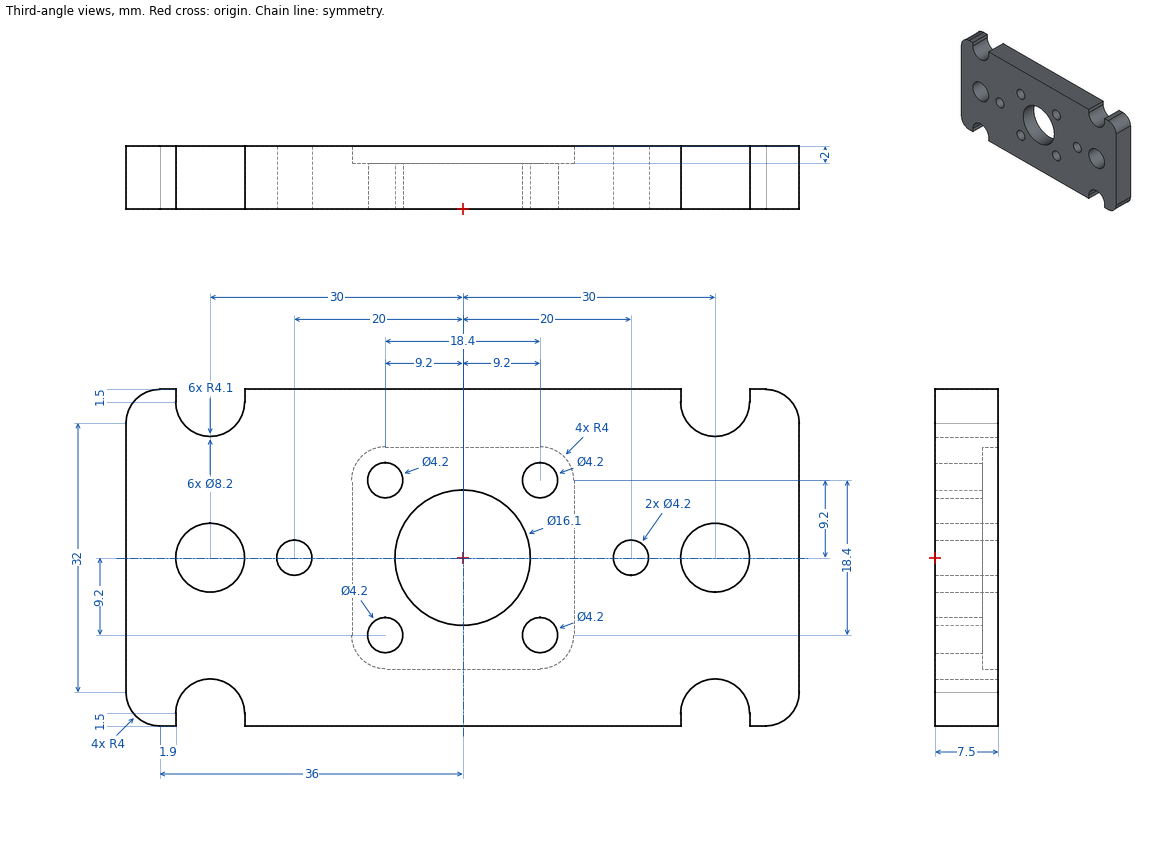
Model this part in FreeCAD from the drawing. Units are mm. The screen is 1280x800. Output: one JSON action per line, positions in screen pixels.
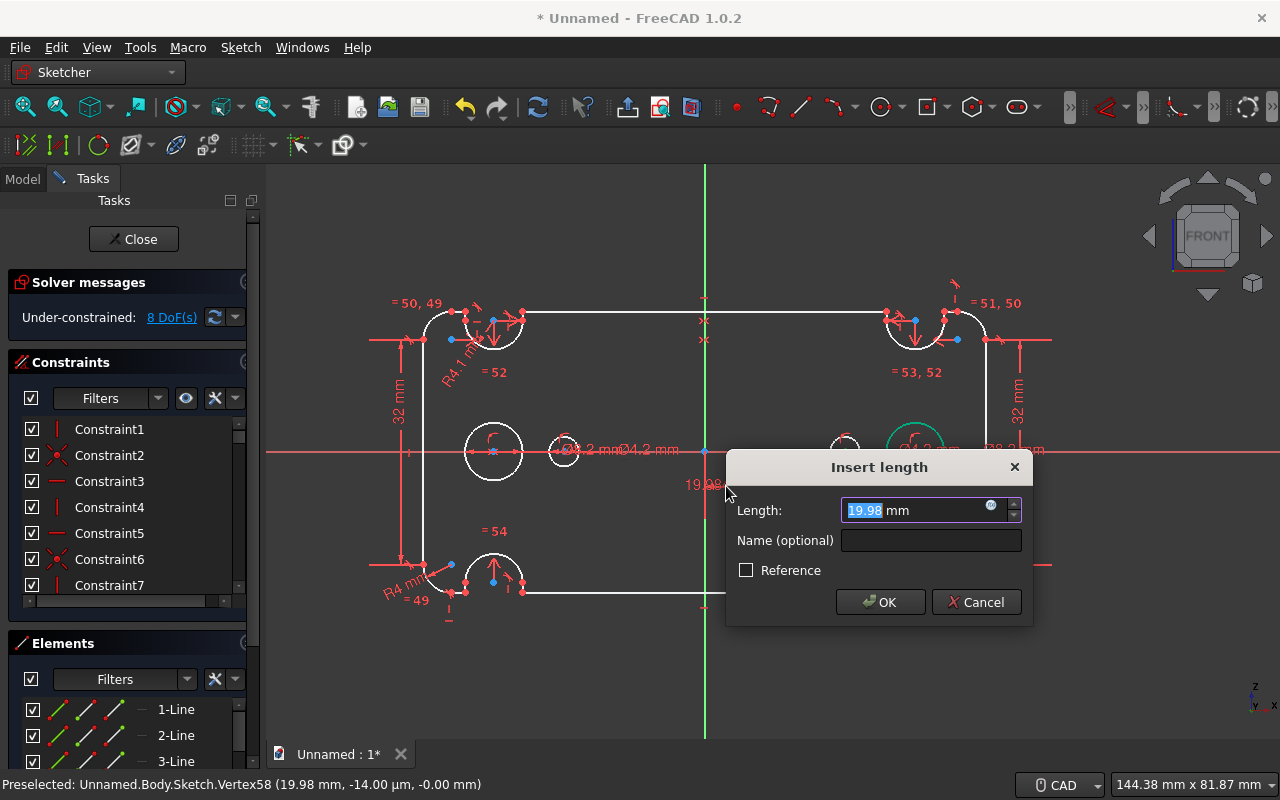
{"action": "type", "text": "20"}
{"action": "key", "text": "Return"}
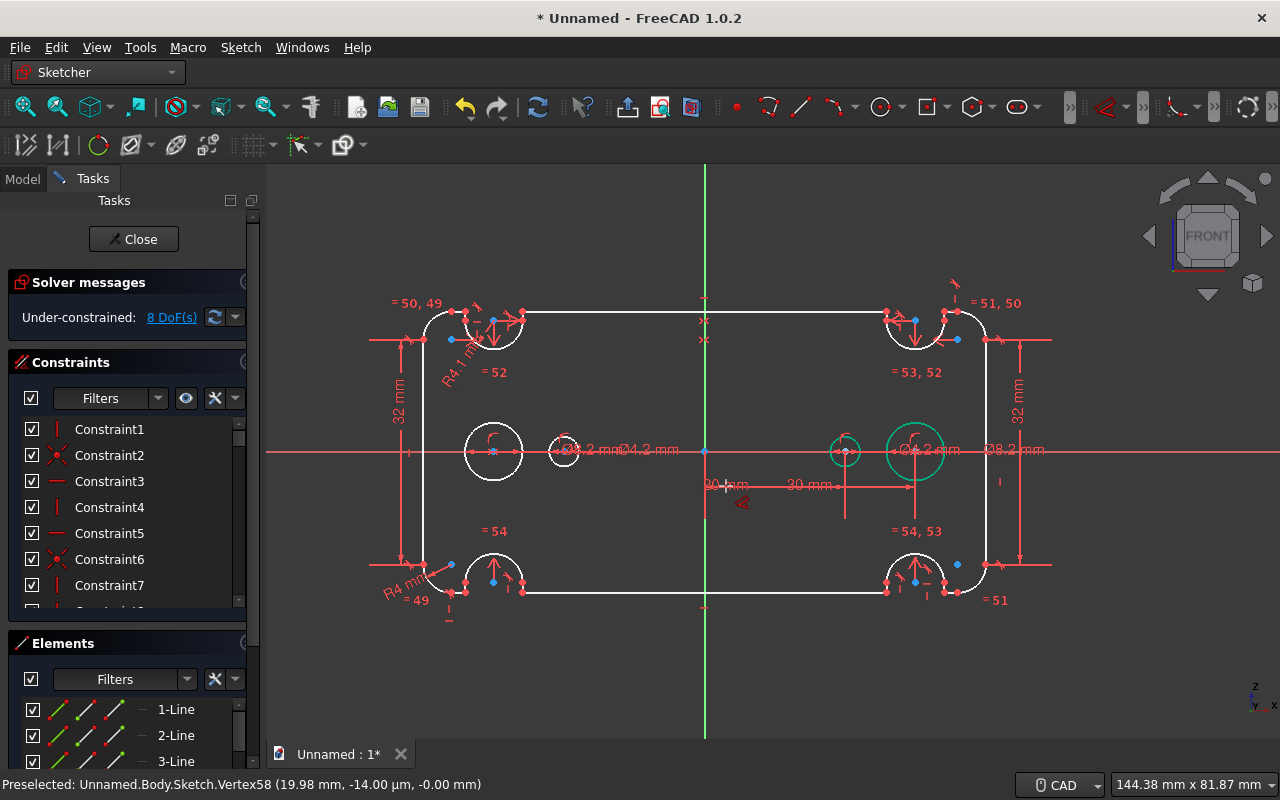
{"action": "left_click", "coordinate": [564, 452]}
{"action": "left_click", "coordinate": [634, 486]}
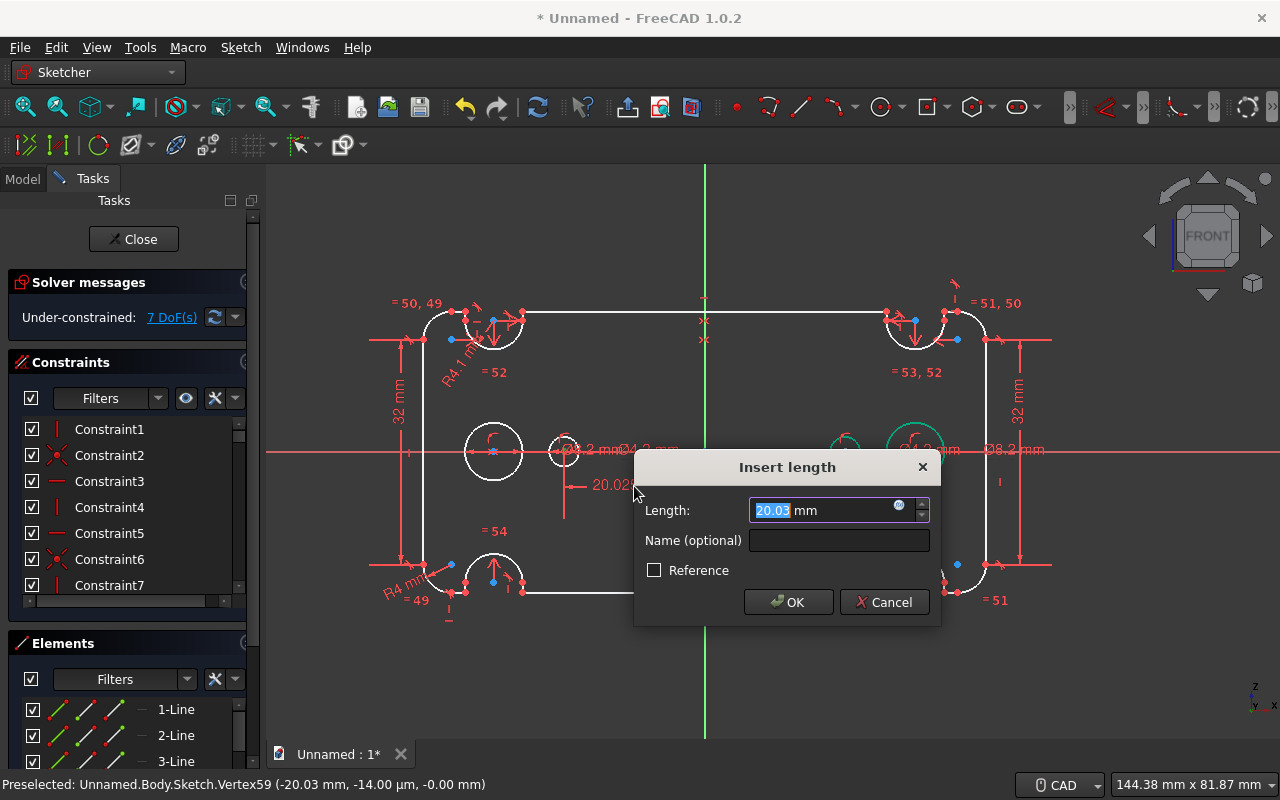
{"action": "type", "text": "20"}
{"action": "key", "text": "Return"}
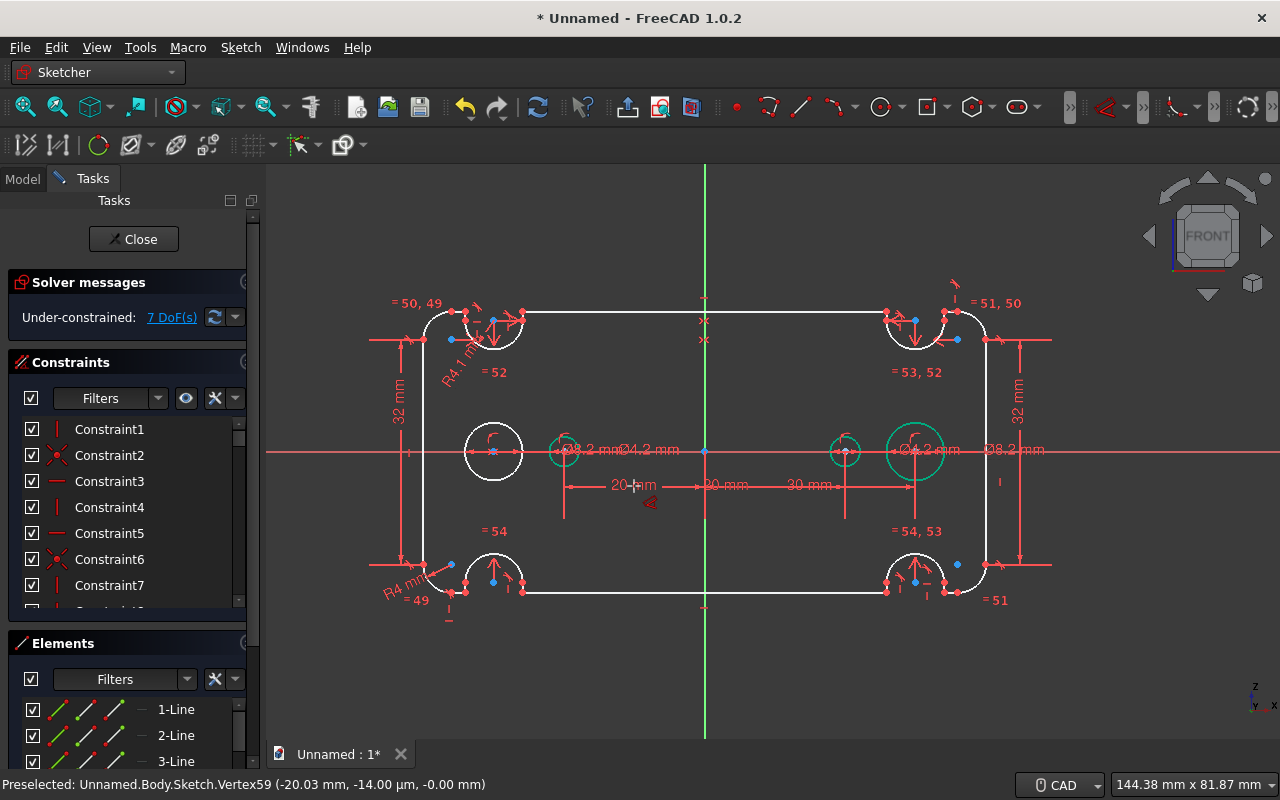
{"action": "left_click", "coordinate": [494, 452]}
{"action": "left_click", "coordinate": [551, 486]}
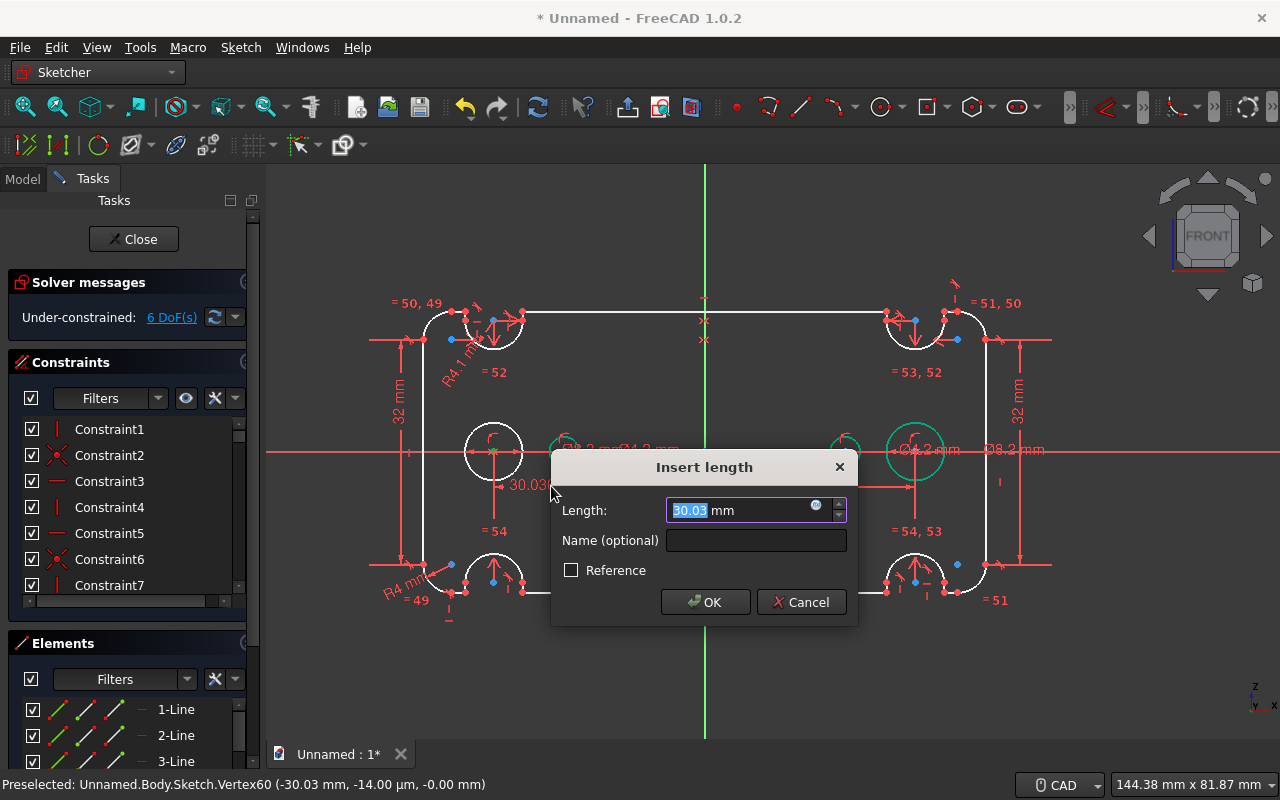
{"action": "type", "text": "30"}
{"action": "key", "text": "Return"}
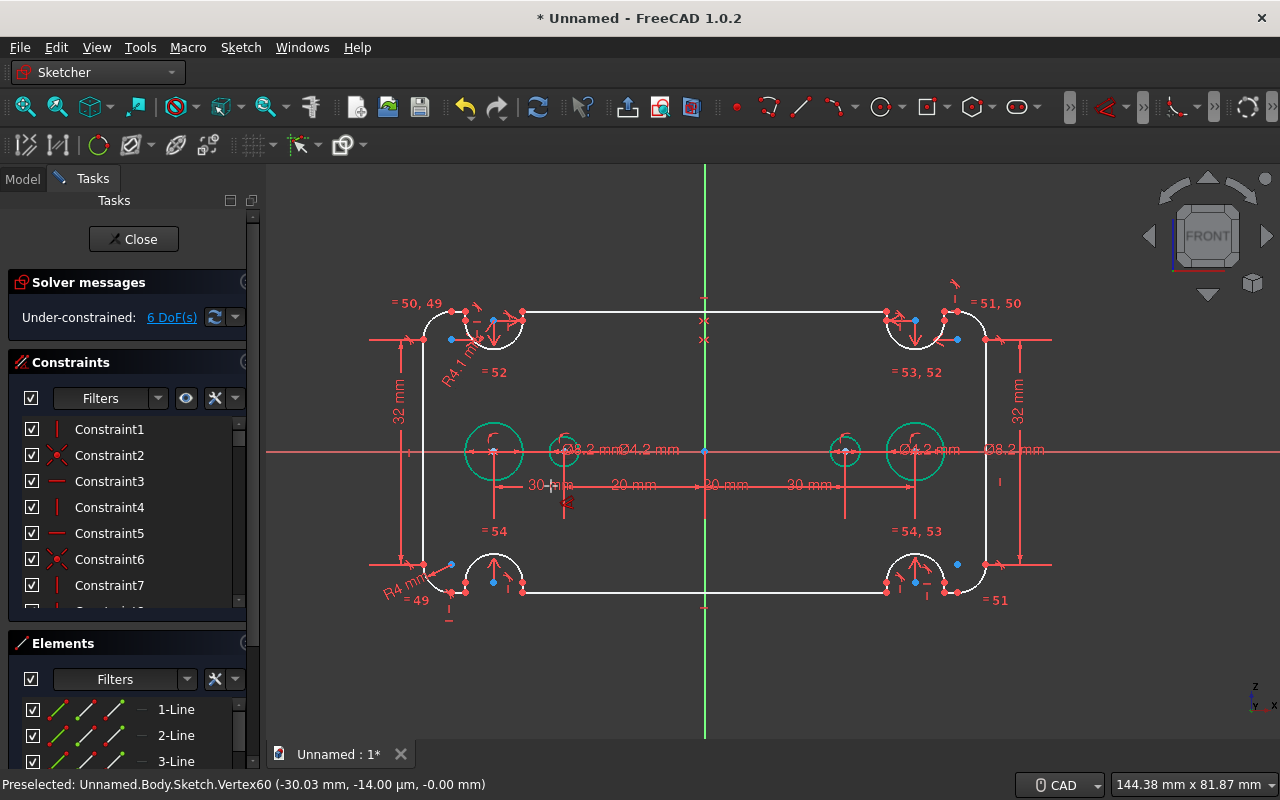
{"action": "scroll", "coordinate": [465, 588], "scroll_direction": "up", "scroll_amount": 7}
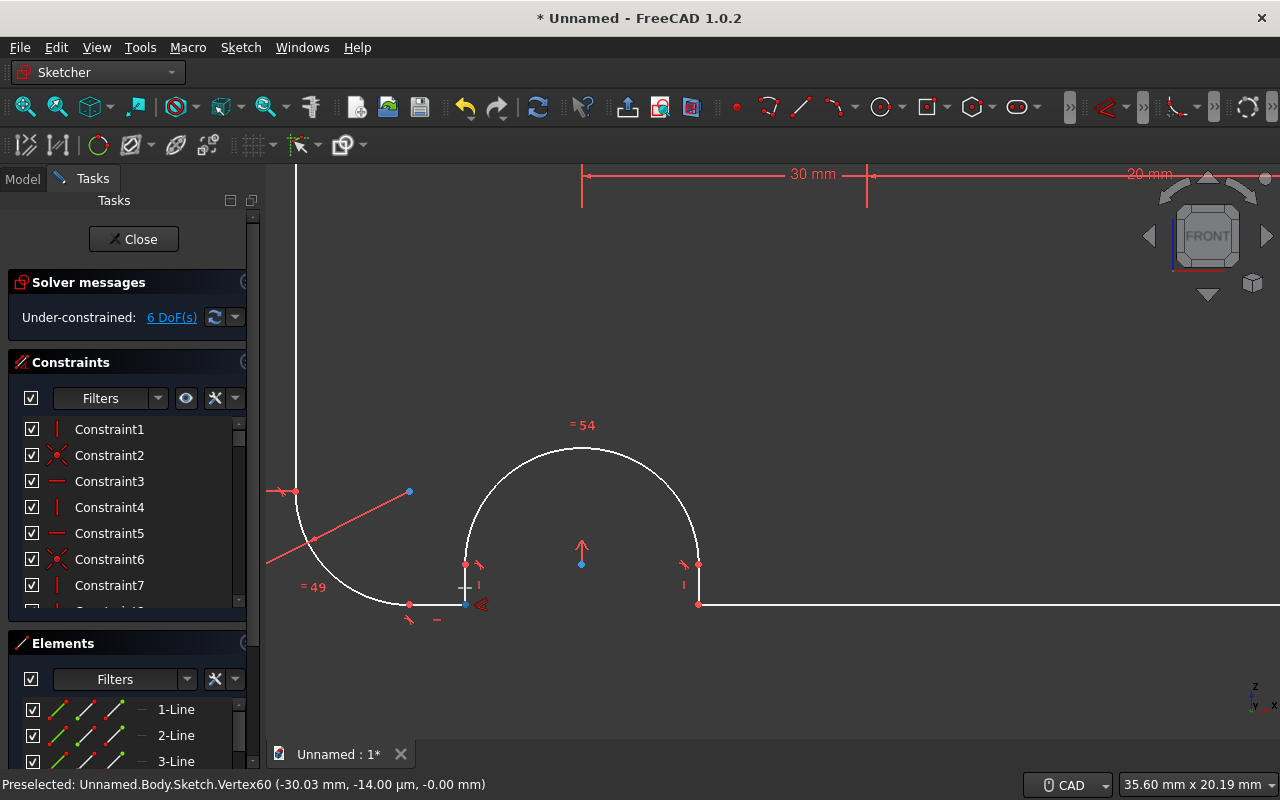
{"action": "left_click", "coordinate": [465, 585]}
{"action": "left_click", "coordinate": [431, 585]}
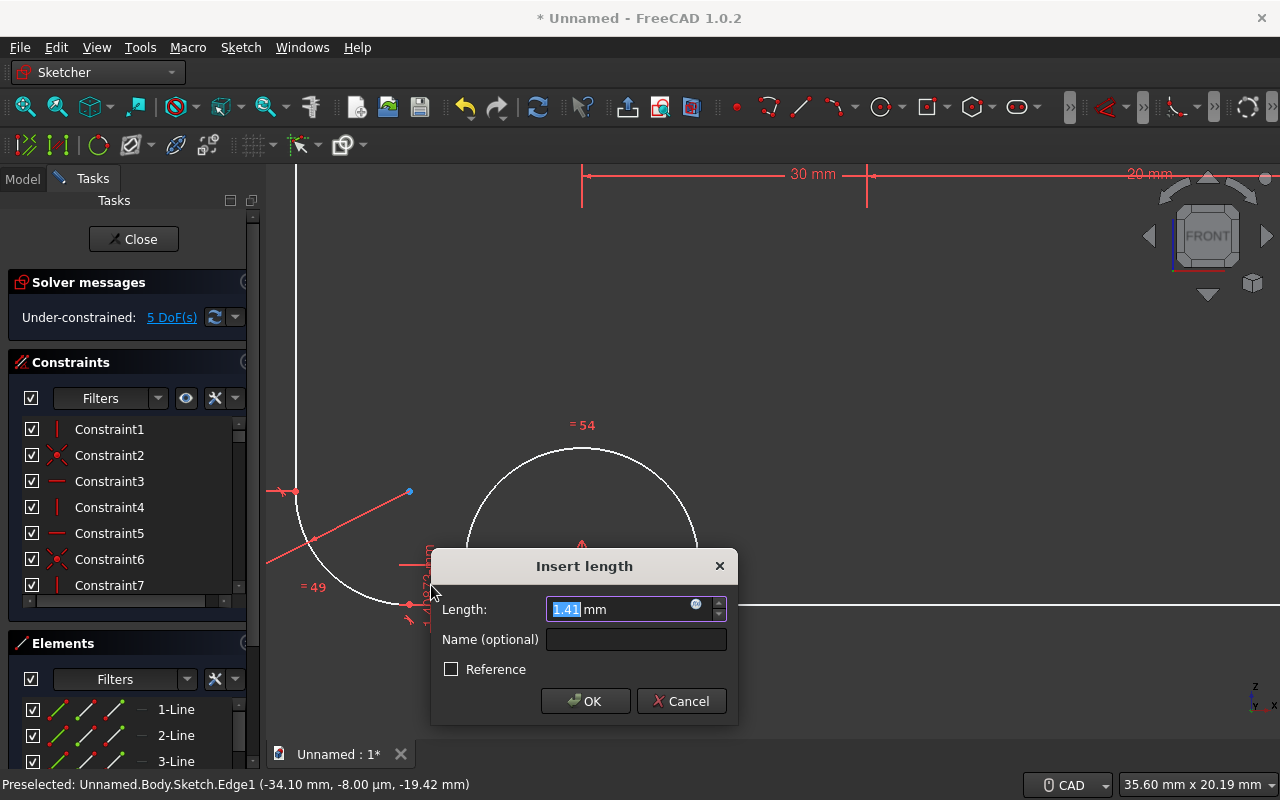
{"action": "type", "text": "1.5"}
{"action": "key", "text": "Return"}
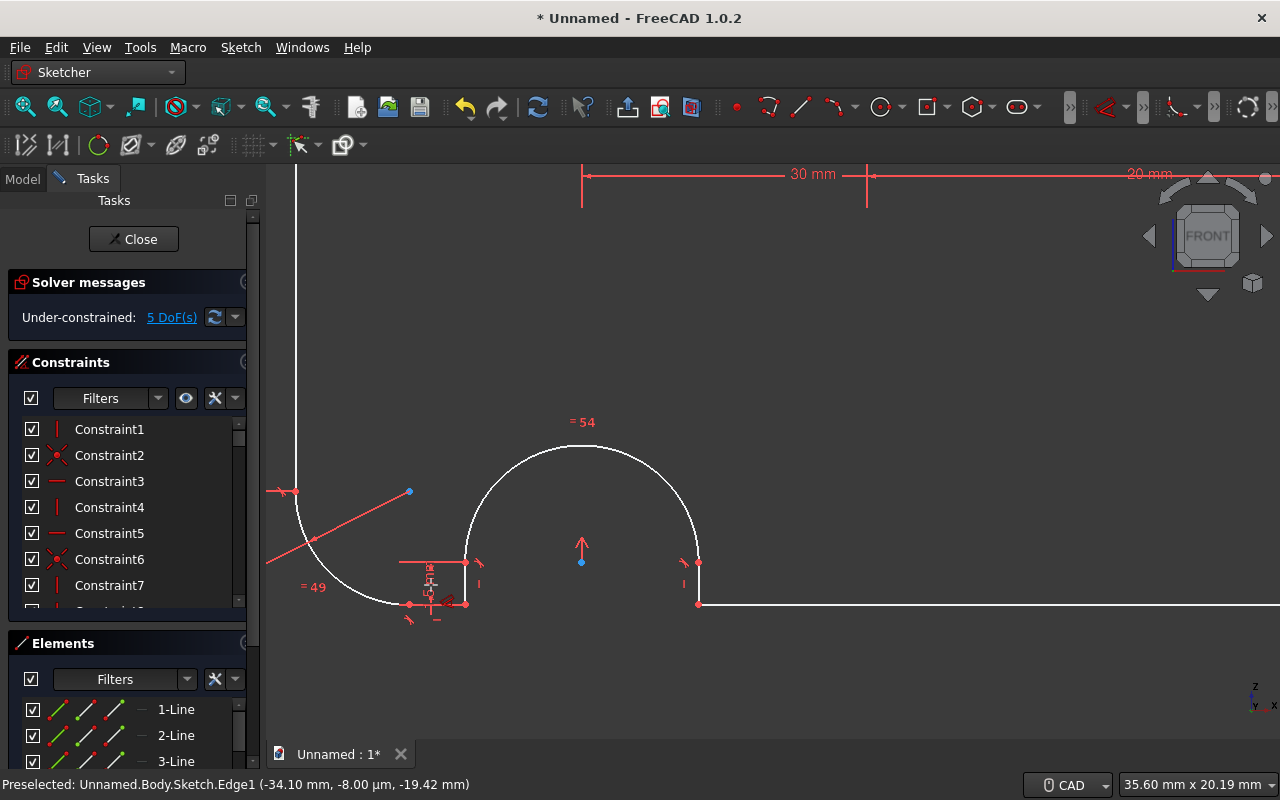
{"action": "left_click", "coordinate": [448, 605]}
{"action": "left_click", "coordinate": [437, 639]}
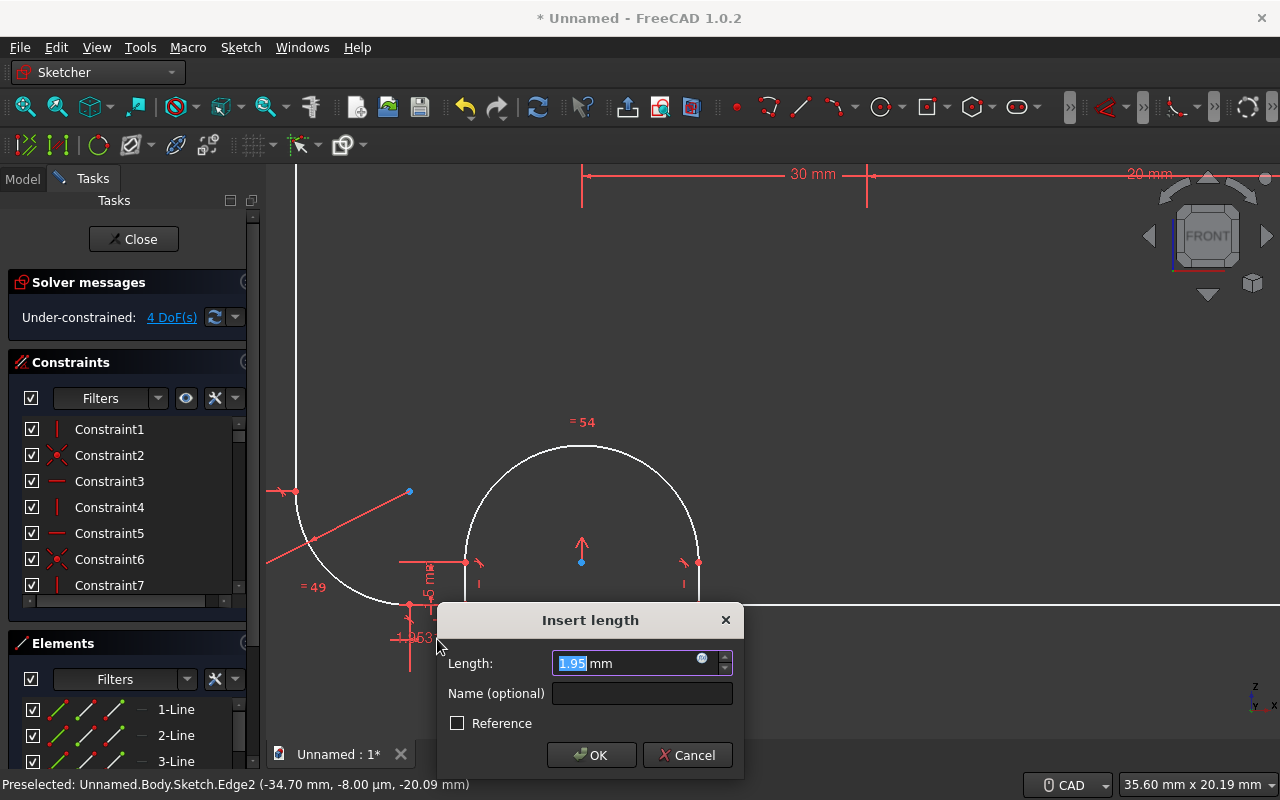
{"action": "type", "text": "1.9"}
{"action": "key", "text": "Return"}